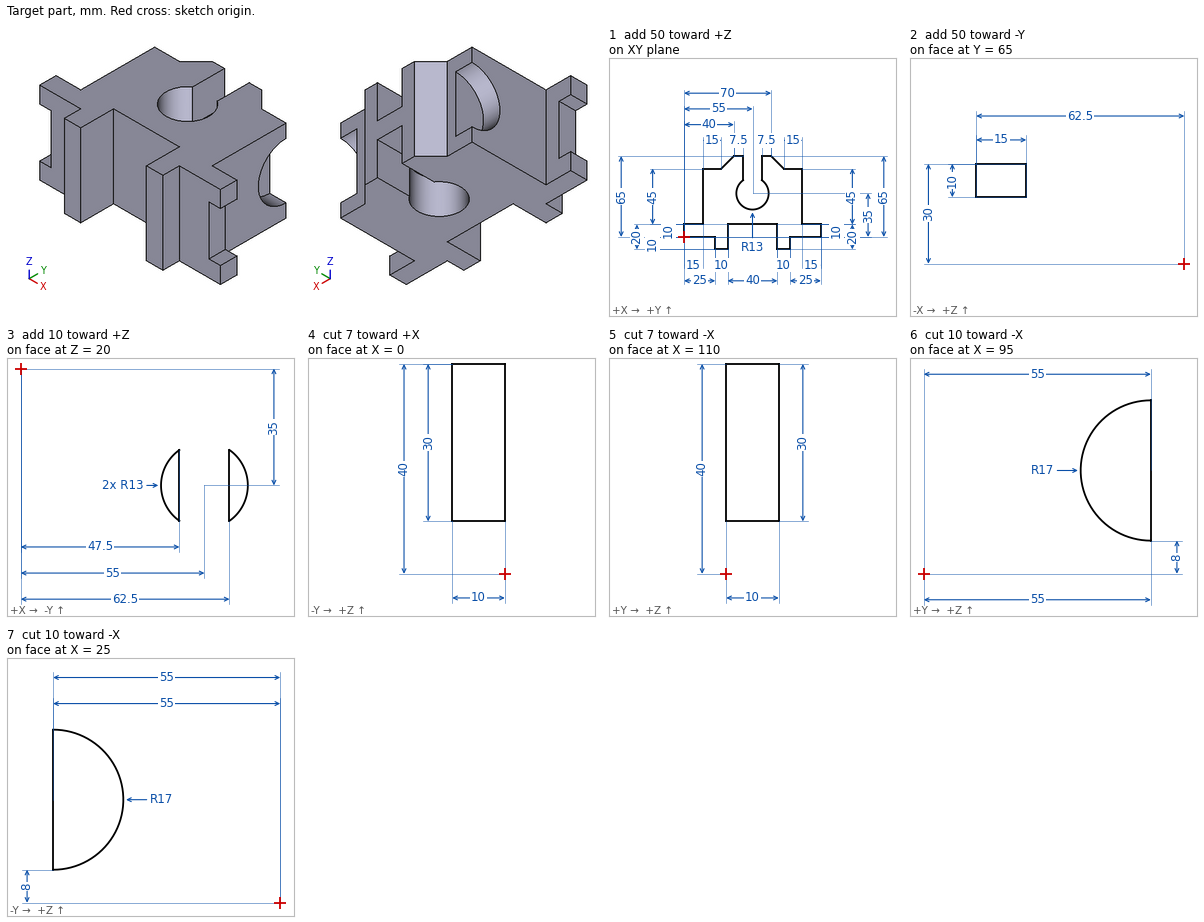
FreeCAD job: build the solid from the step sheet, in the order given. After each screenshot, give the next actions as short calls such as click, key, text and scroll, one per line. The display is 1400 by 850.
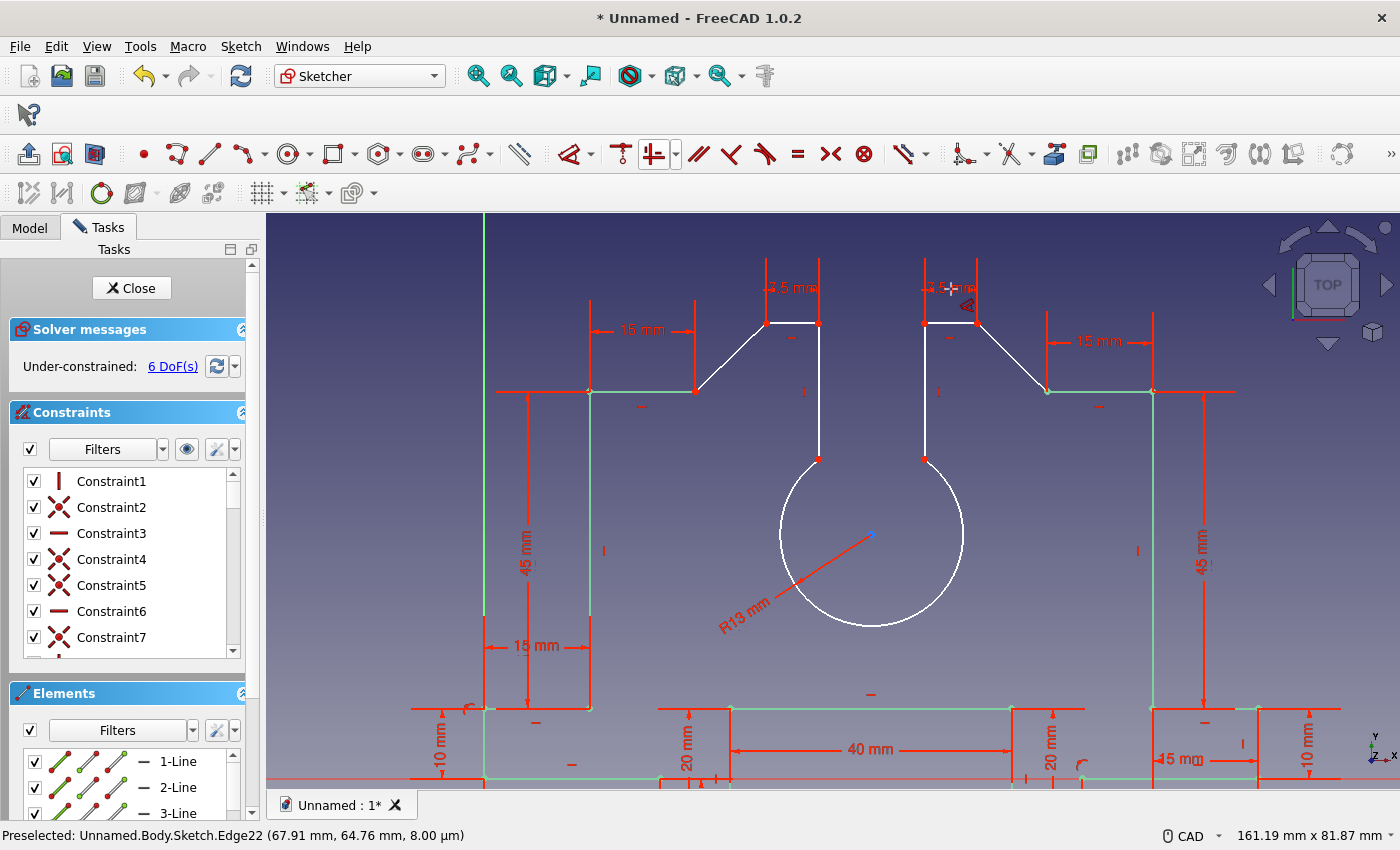
click(819, 323)
click(450, 542)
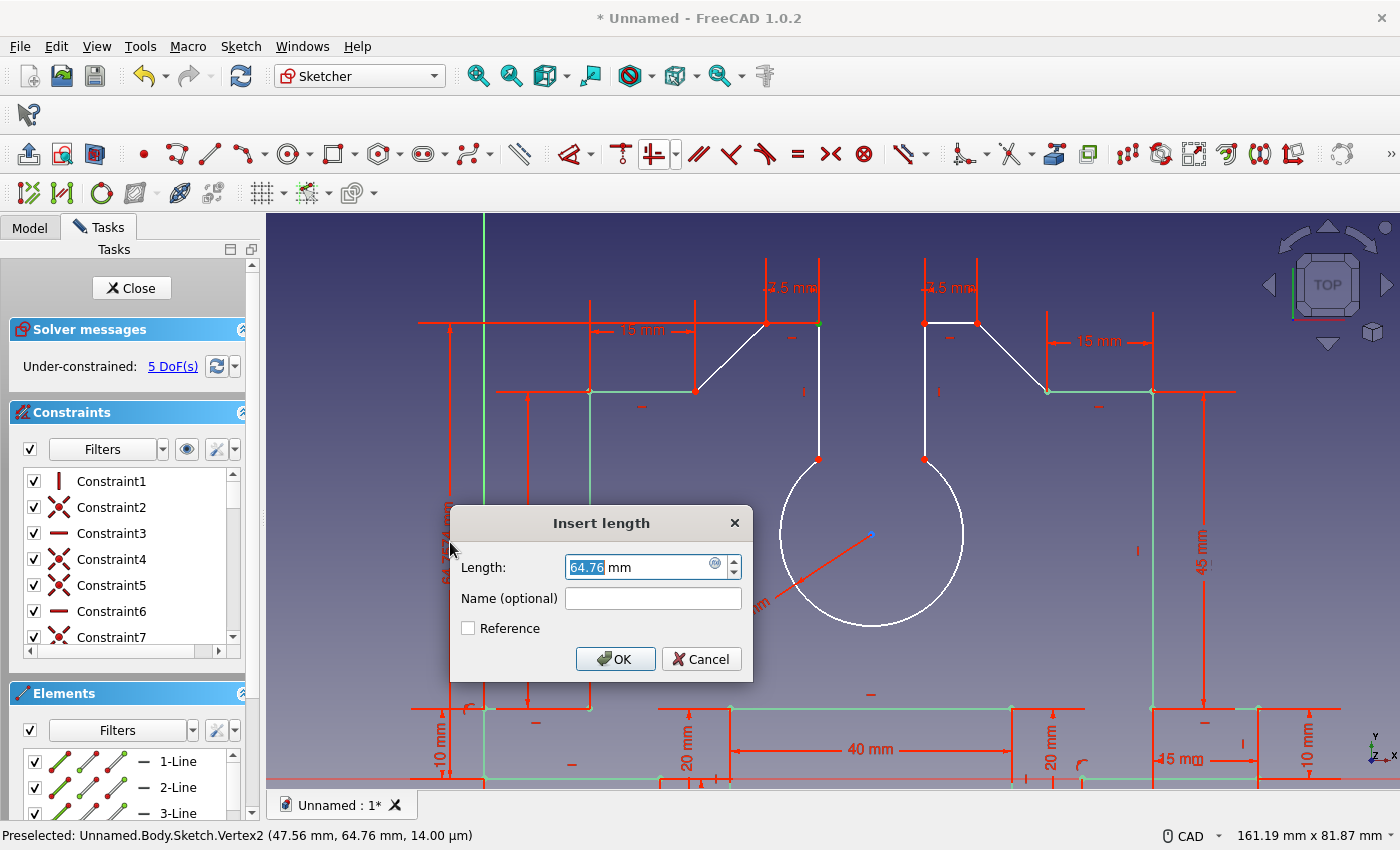
text(65)
key(Return)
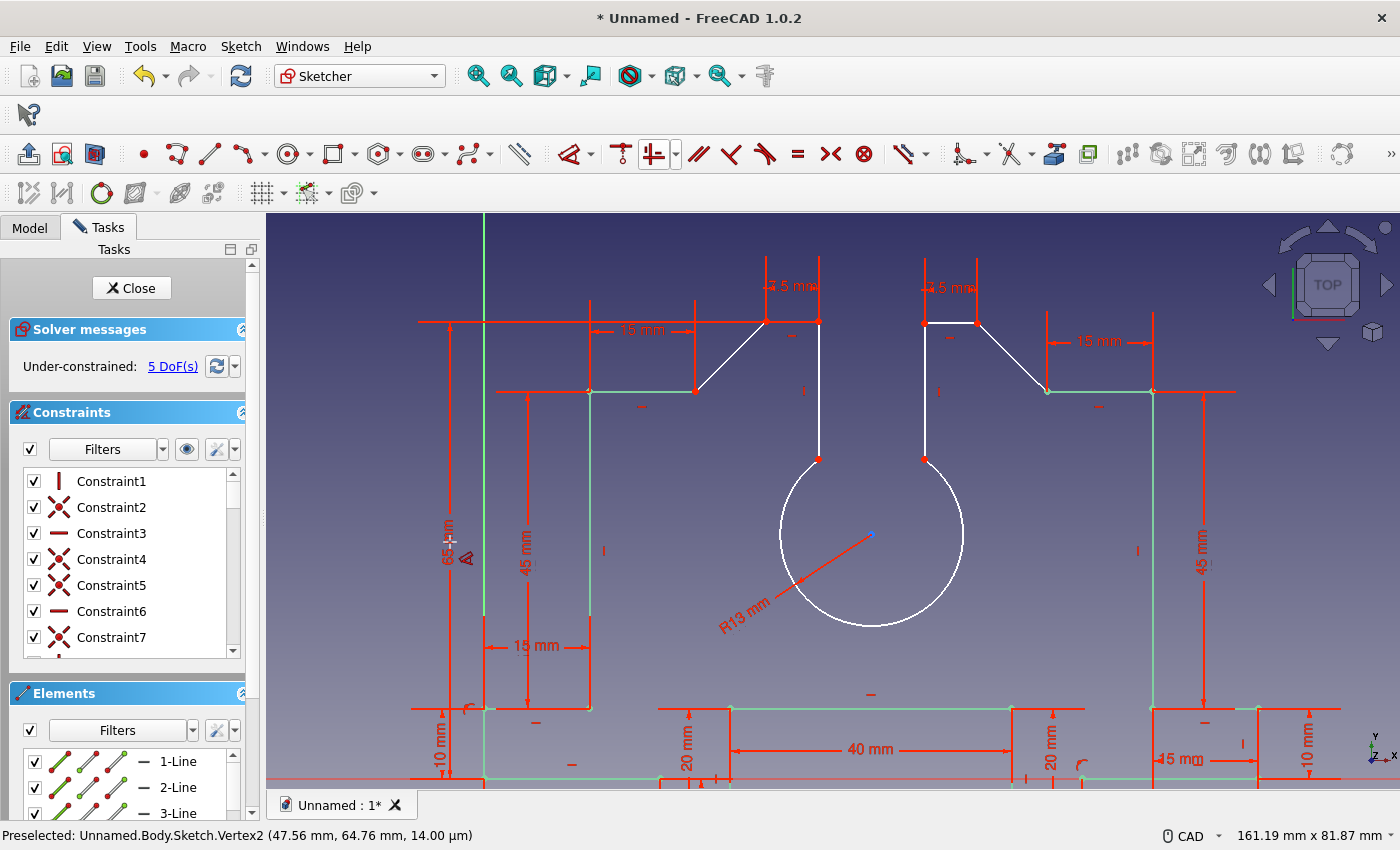
click(766, 322)
click(625, 288)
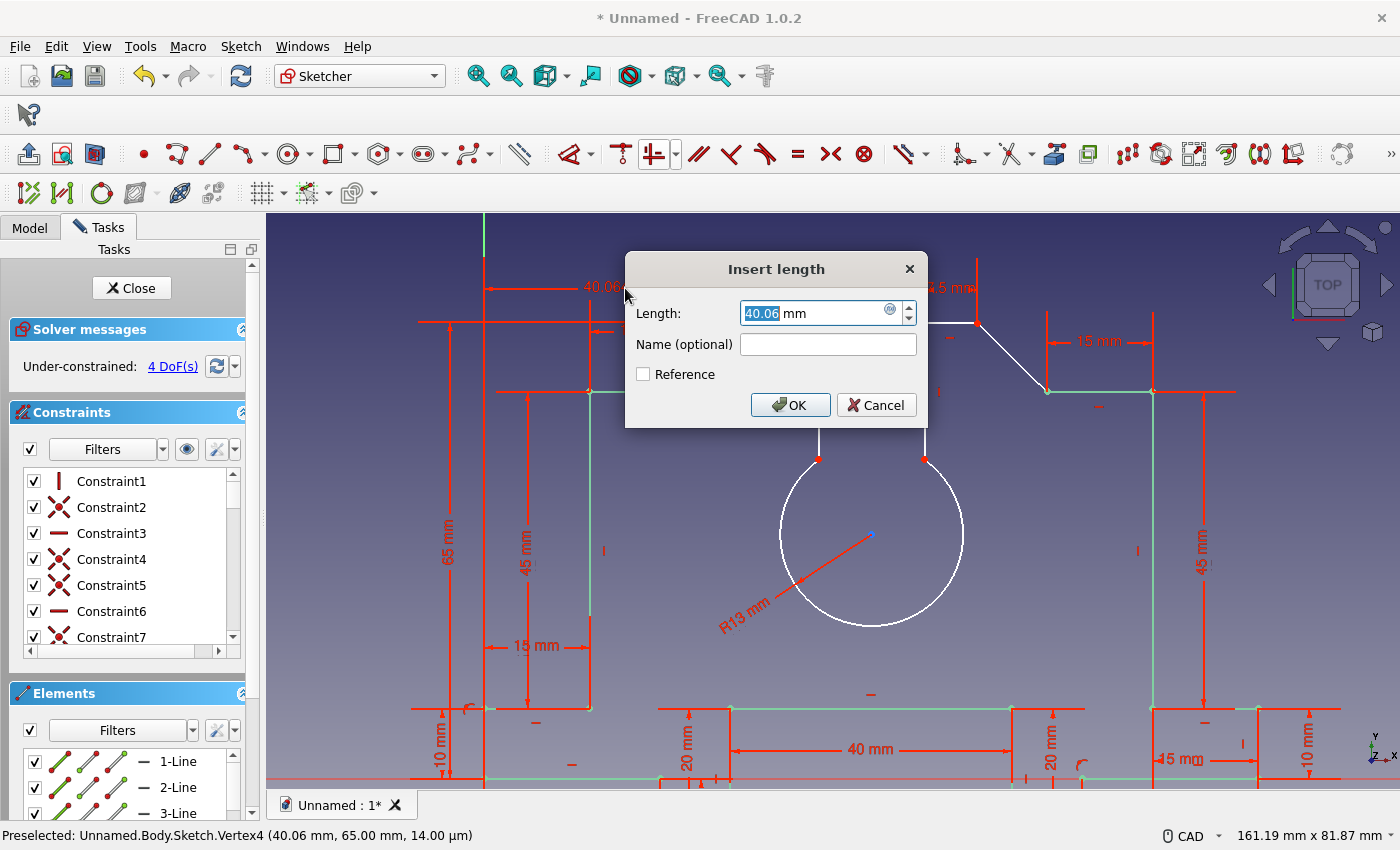
text(40)
key(Return)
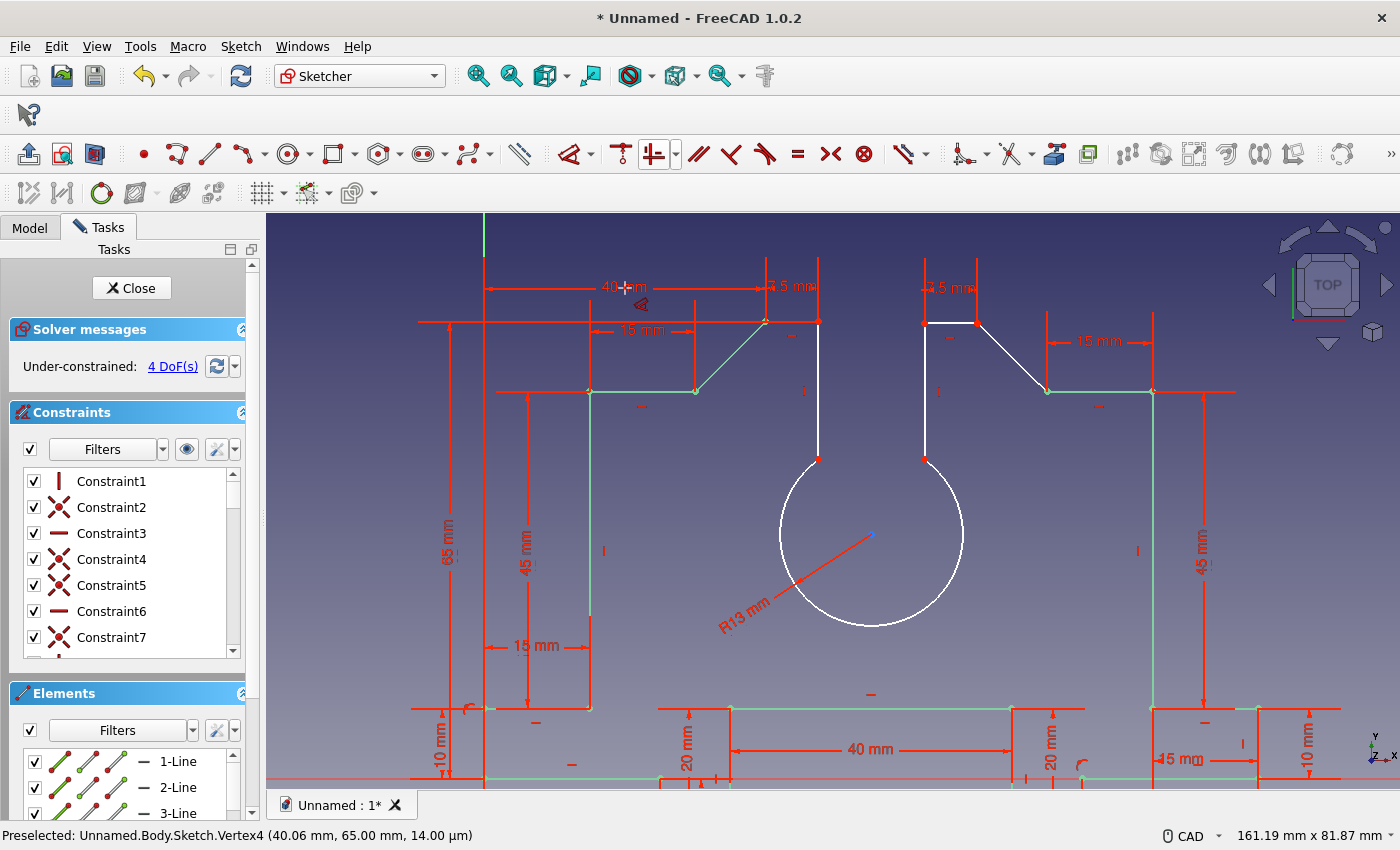
click(977, 323)
click(731, 265)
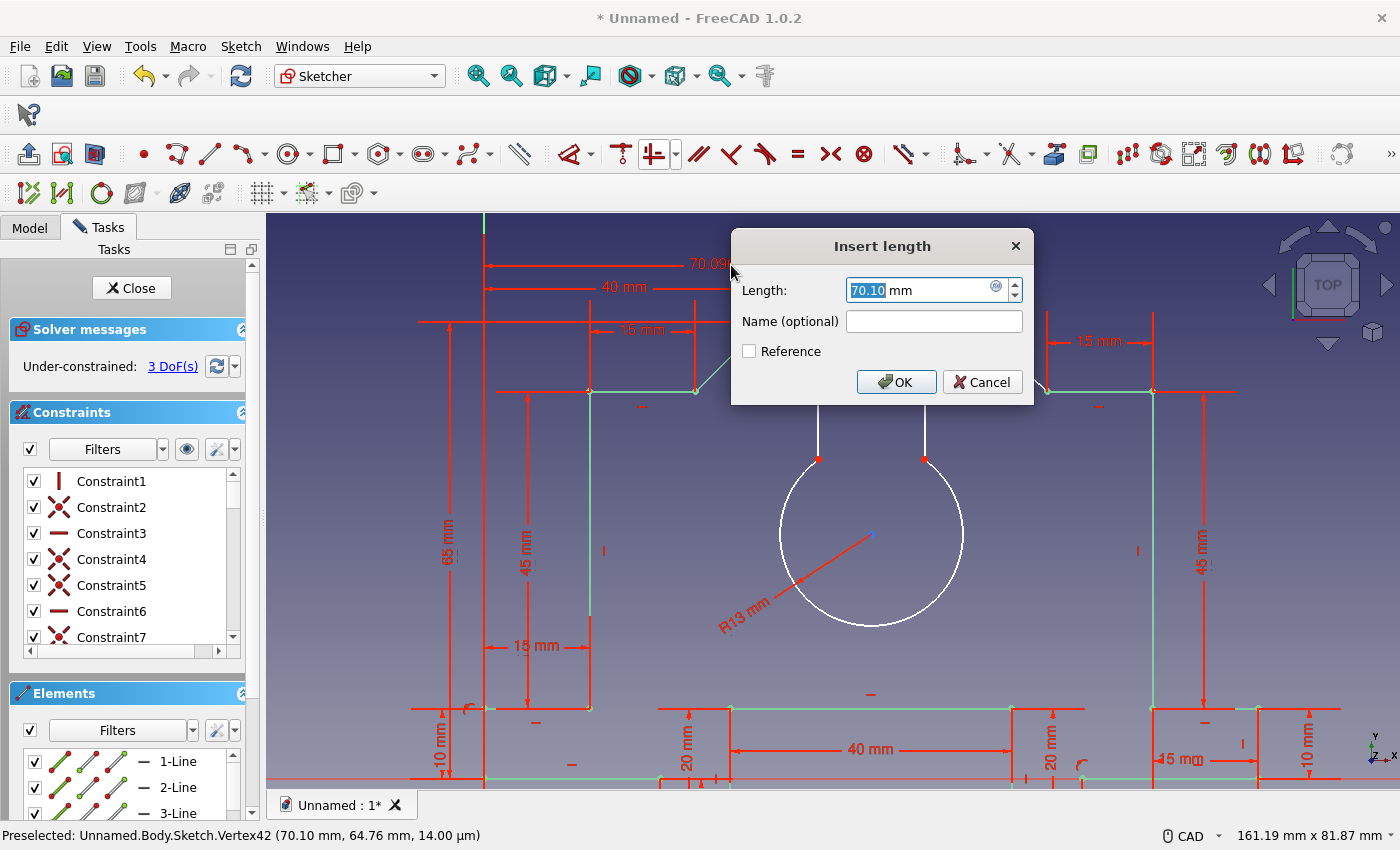
text(70)
key(Return)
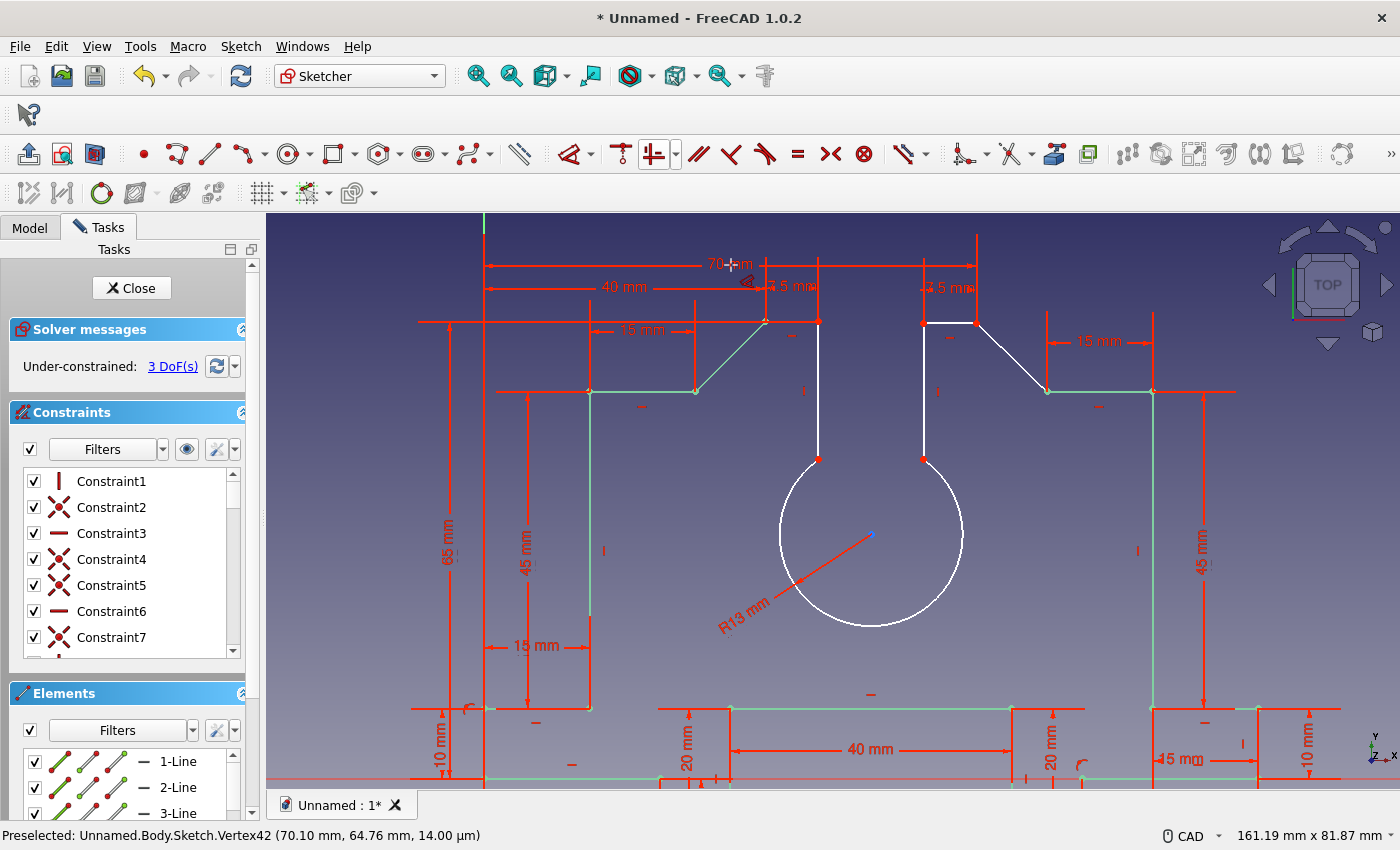
click(977, 323)
click(450, 441)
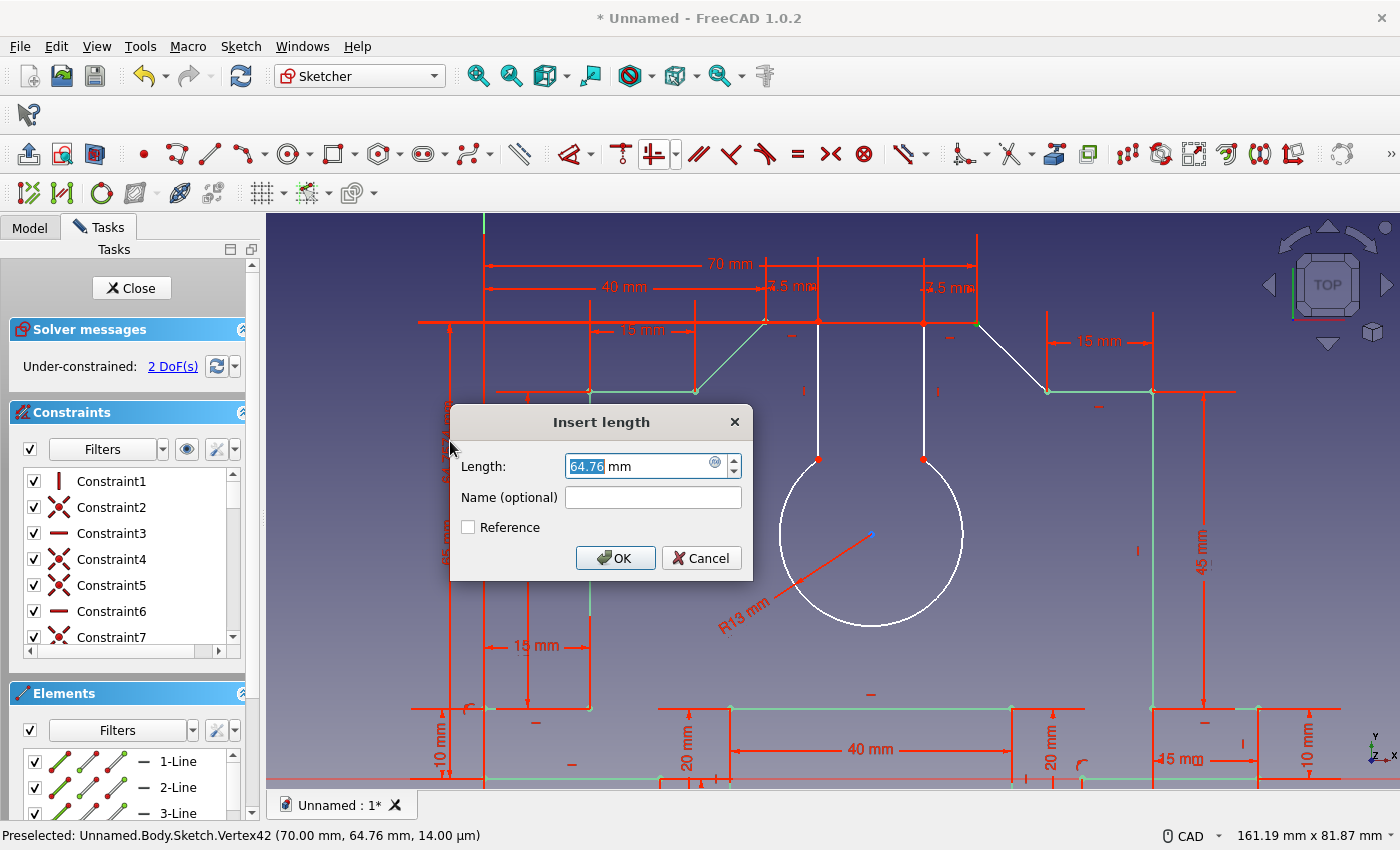
text(65)
key(Return)